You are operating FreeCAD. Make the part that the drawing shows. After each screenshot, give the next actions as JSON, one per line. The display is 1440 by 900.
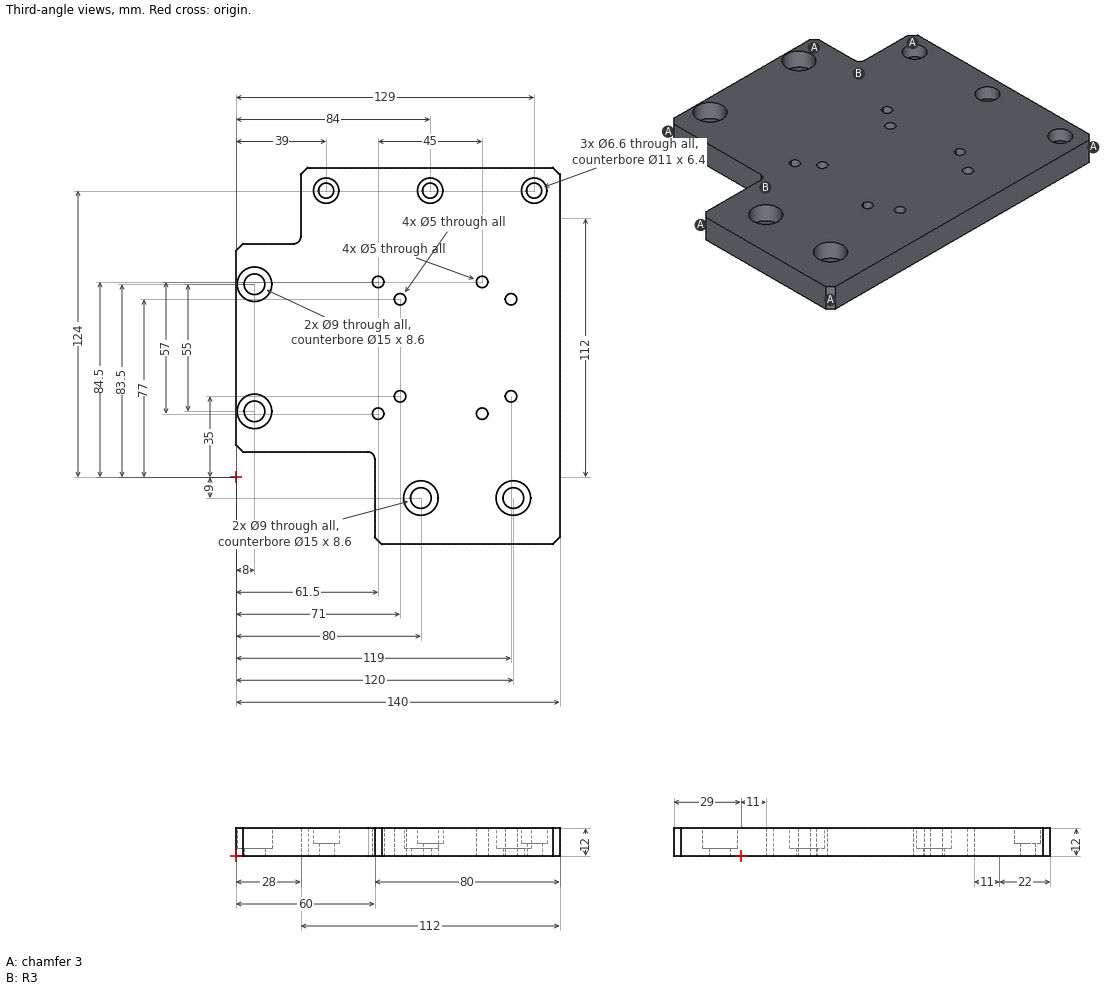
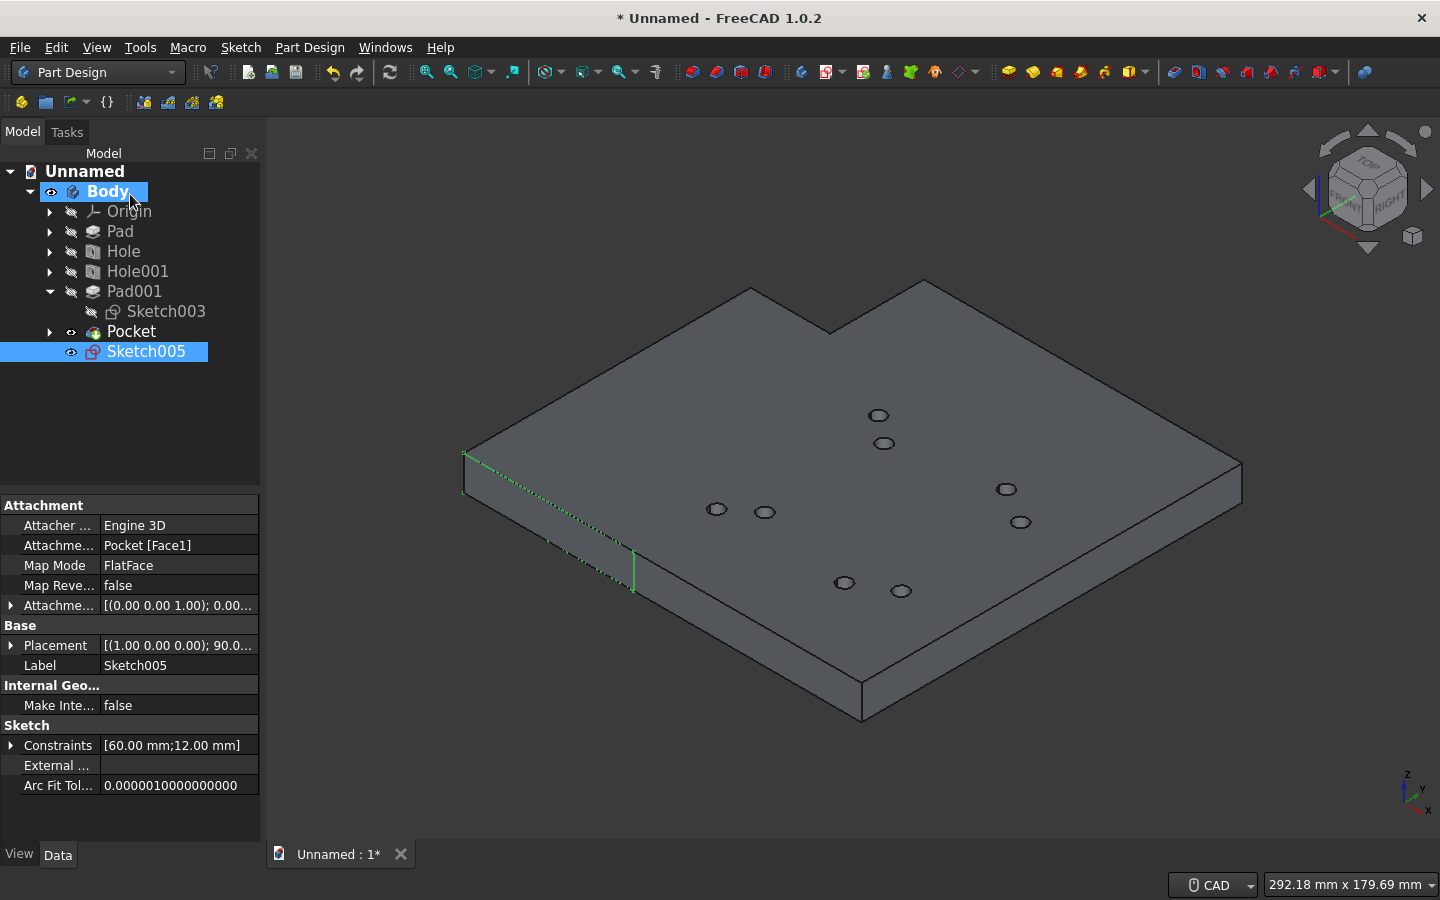
{"action": "left_click", "coordinate": [1176, 72]}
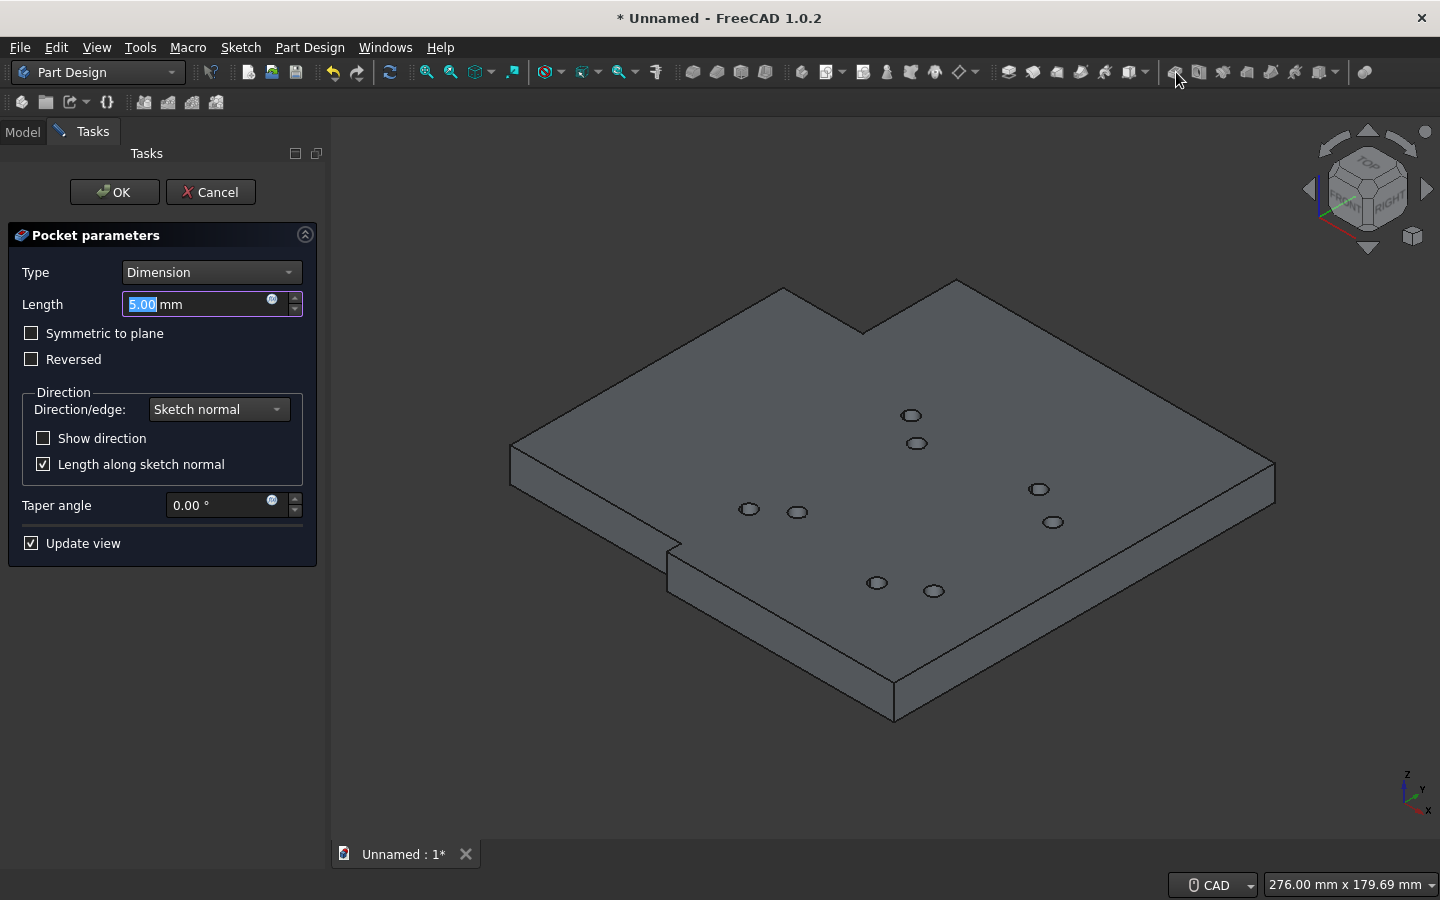
{"action": "type", "text": "11"}
{"action": "key", "text": "Tab"}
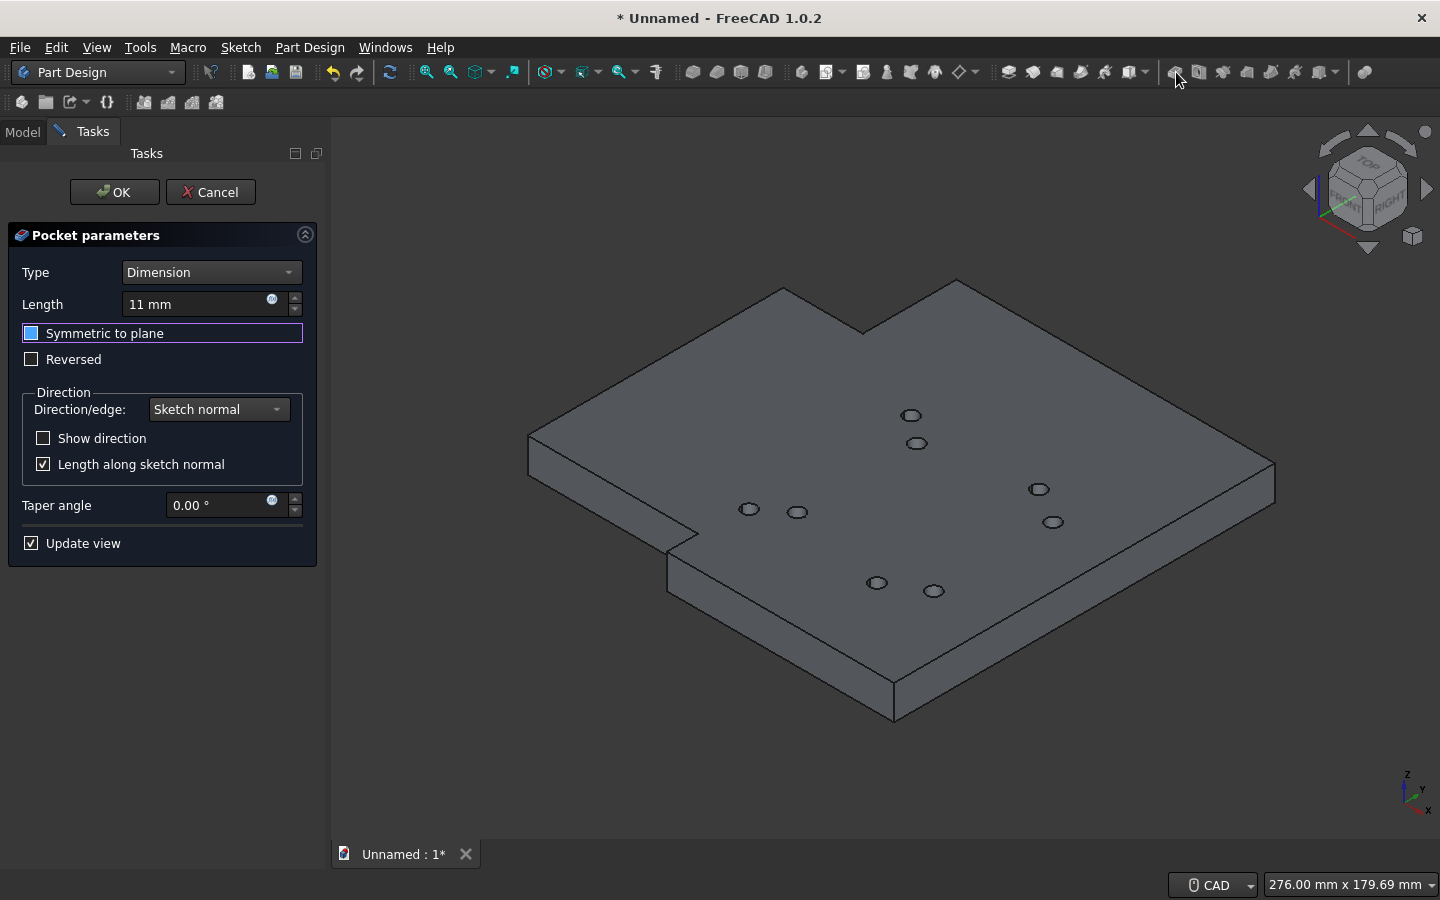
{"action": "left_click", "coordinate": [115, 192]}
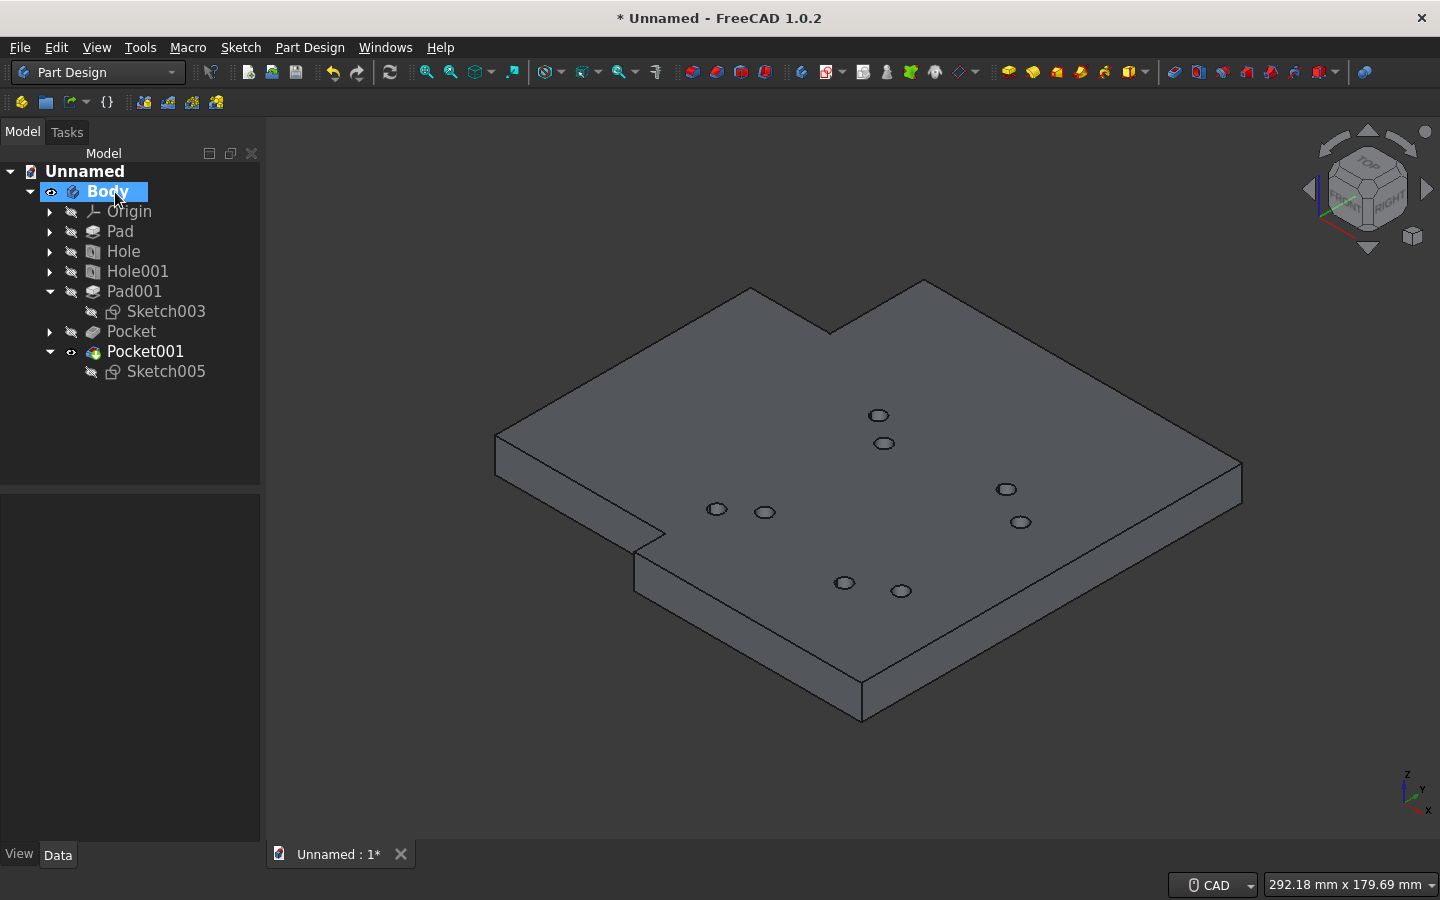
{"action": "left_click", "coordinate": [739, 392]}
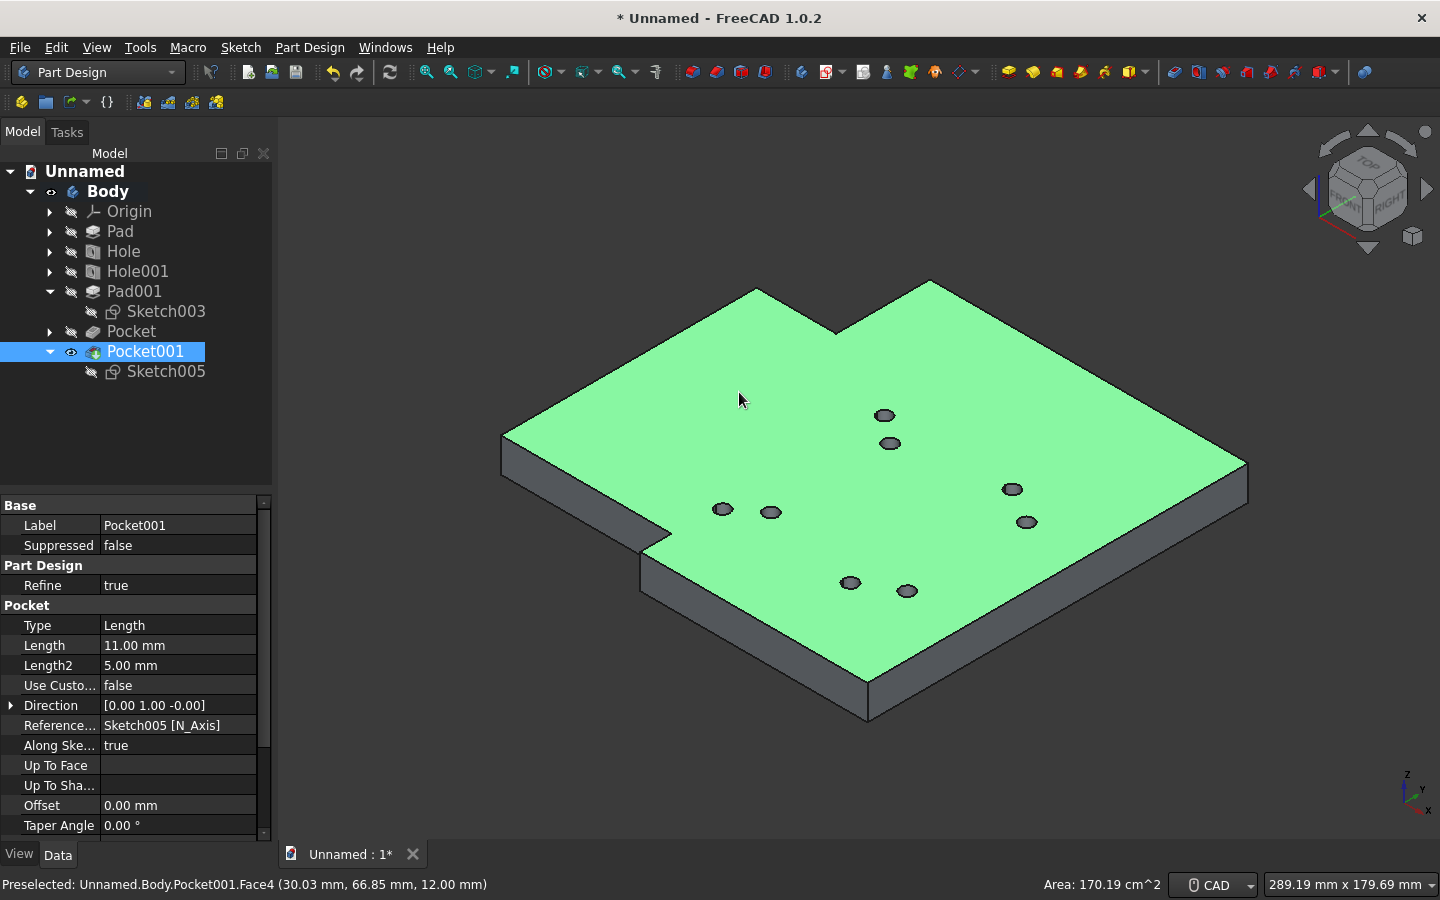
{"action": "left_click", "coordinate": [826, 72]}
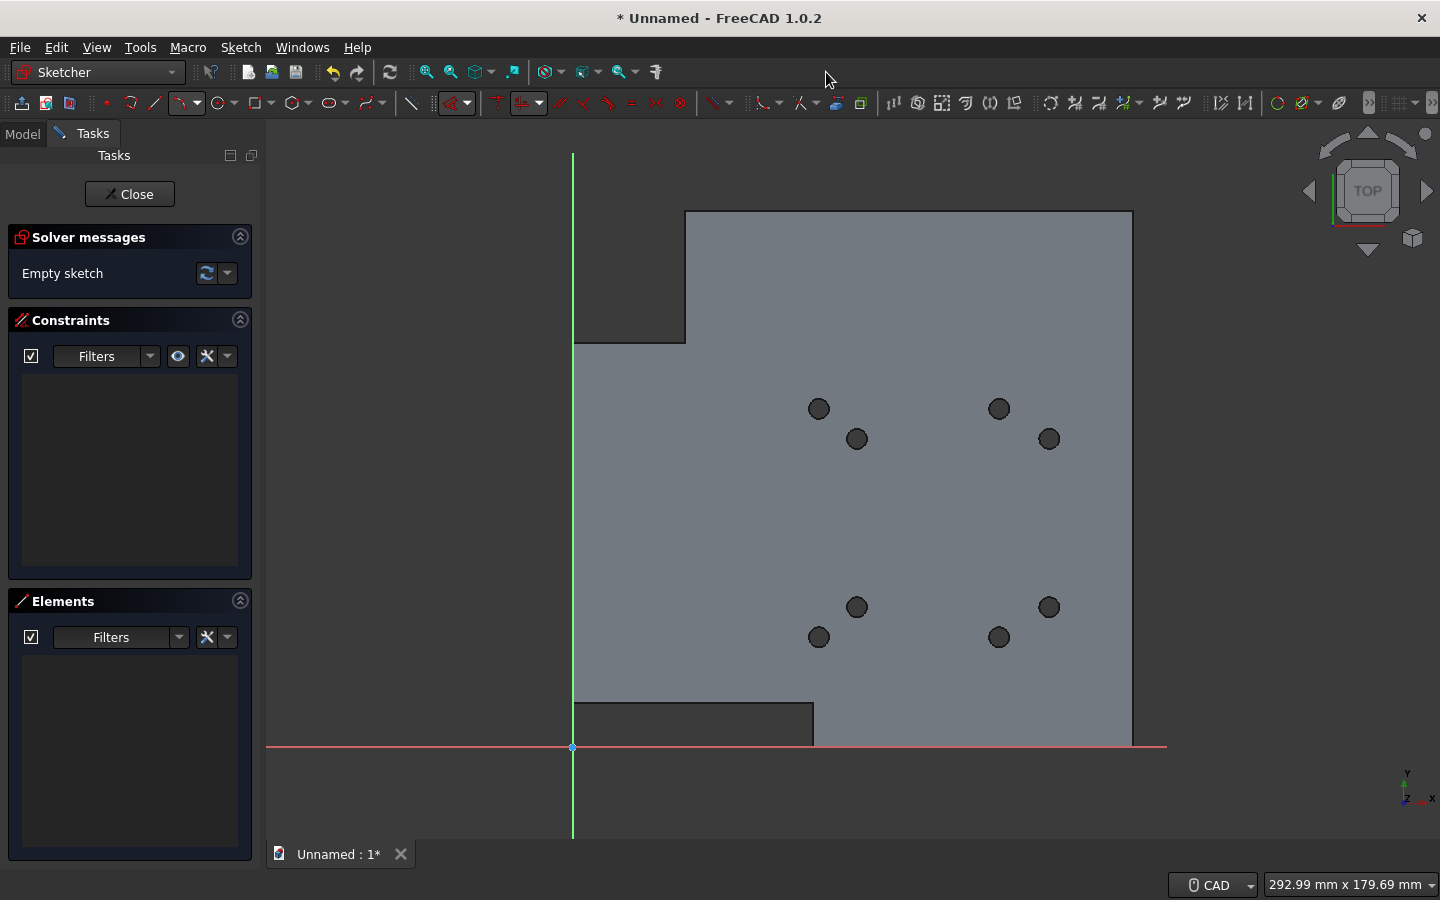
{"action": "key", "text": "g c"}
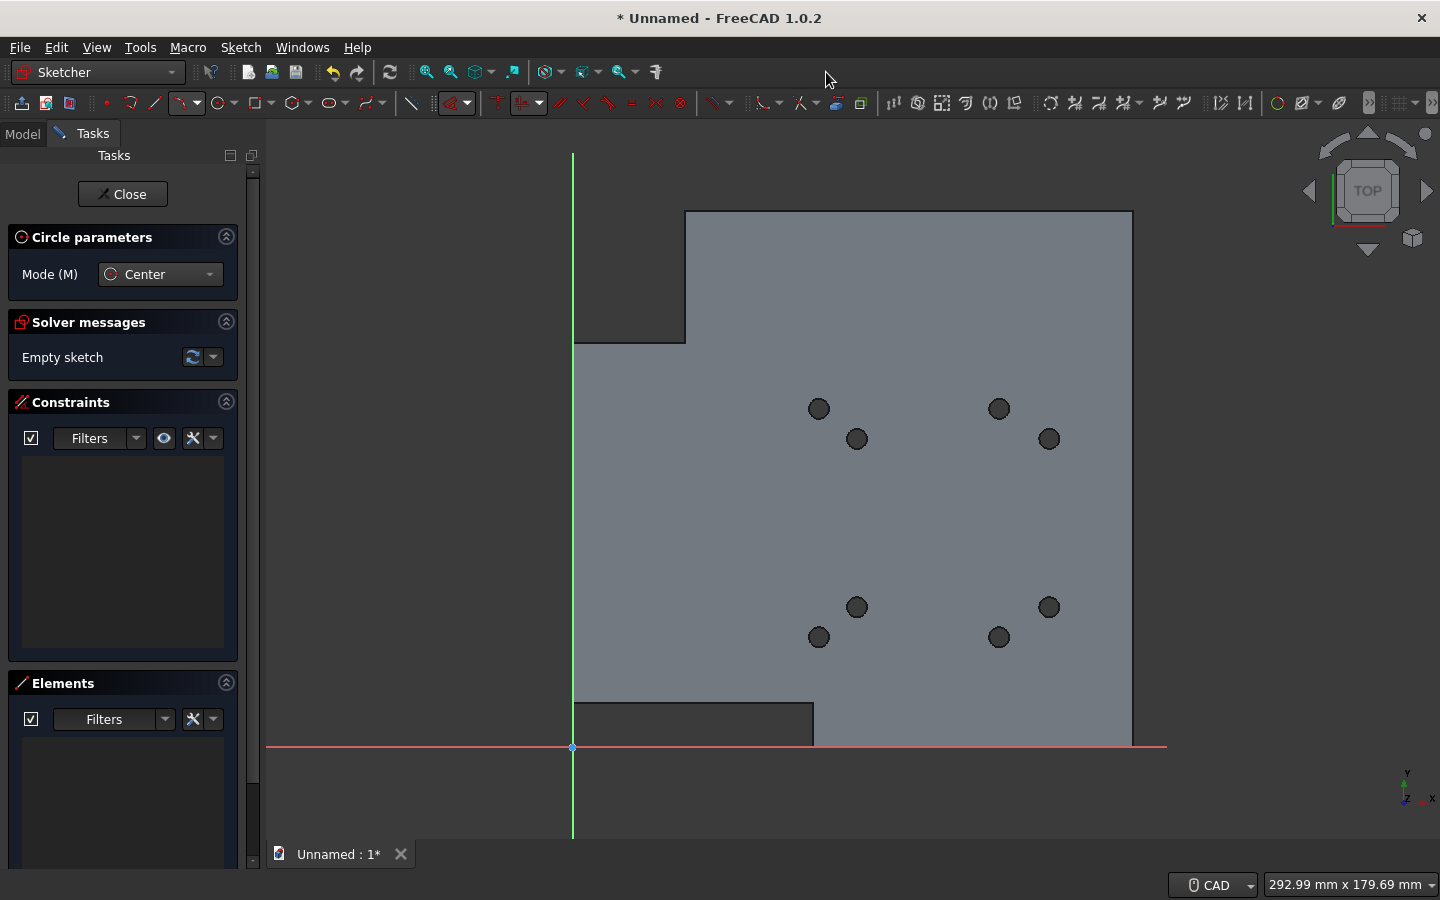
{"action": "scroll", "coordinate": [1089, 251], "scroll_direction": "up", "scroll_amount": 3}